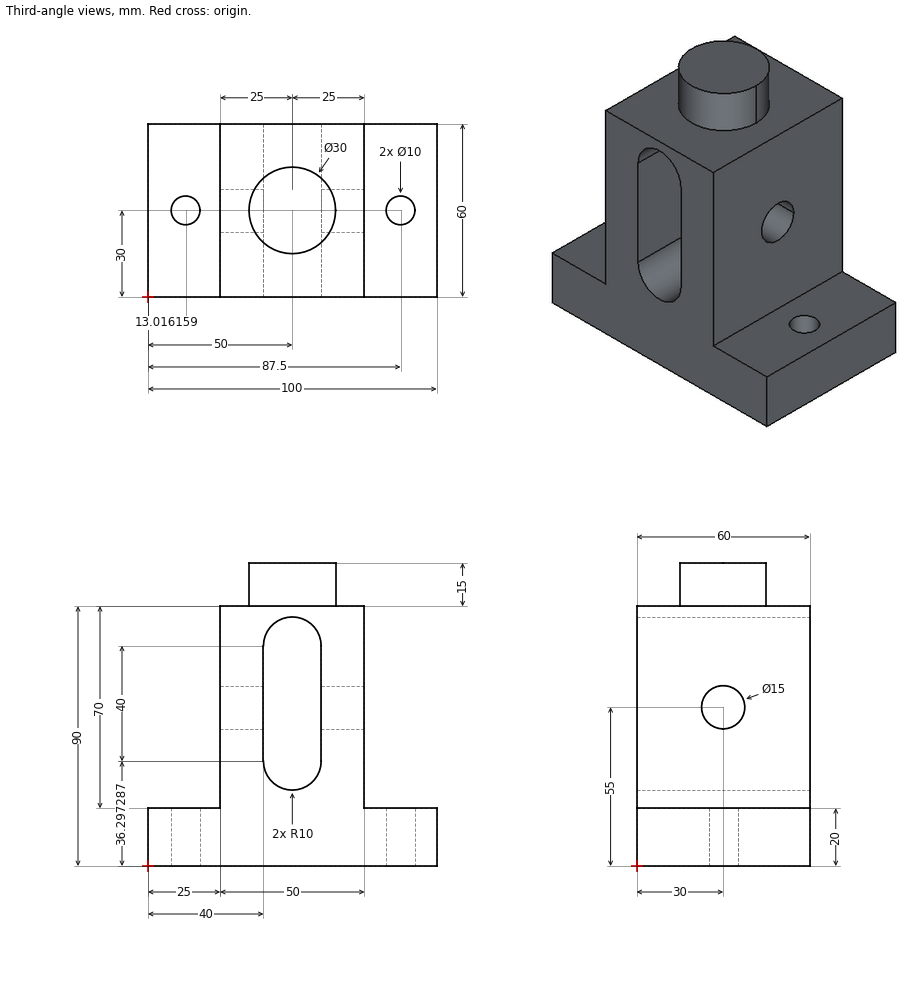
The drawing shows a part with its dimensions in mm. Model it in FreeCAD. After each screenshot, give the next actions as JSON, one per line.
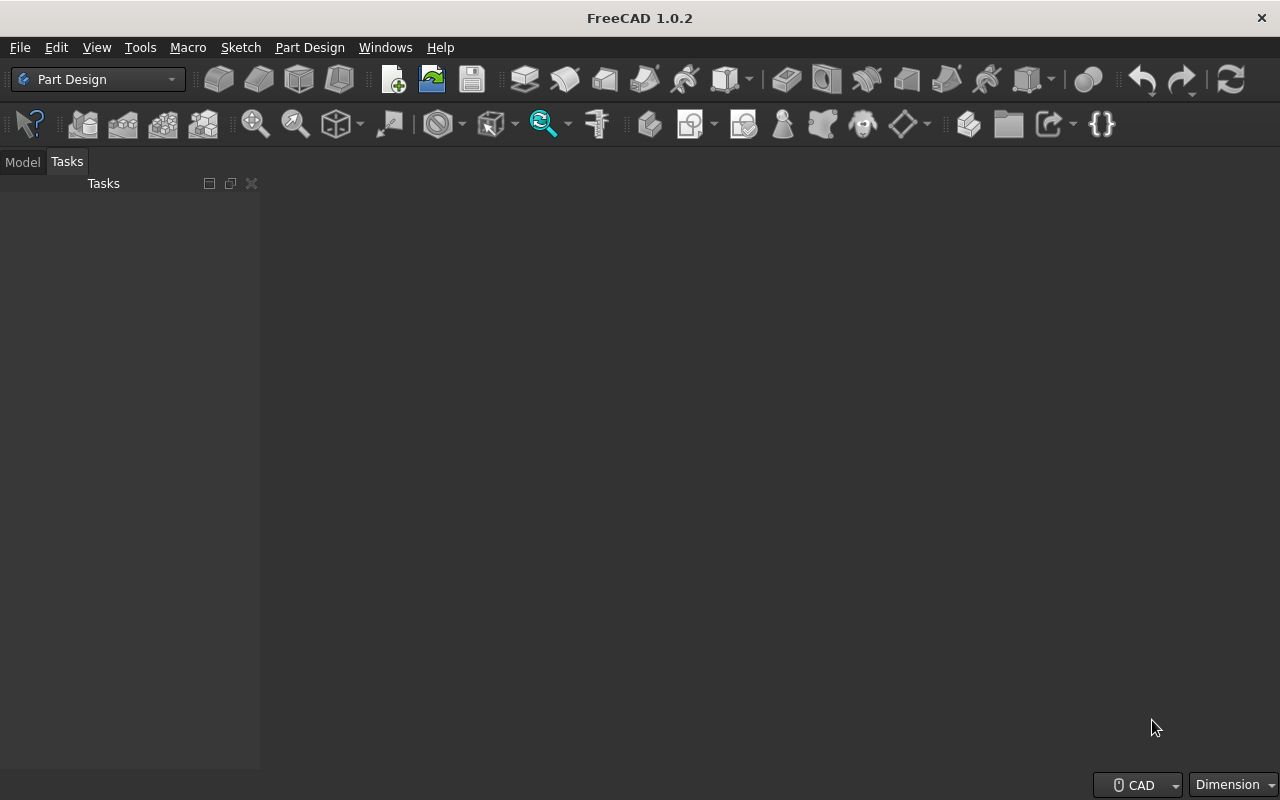
{"action": "left_click", "coordinate": [392, 80]}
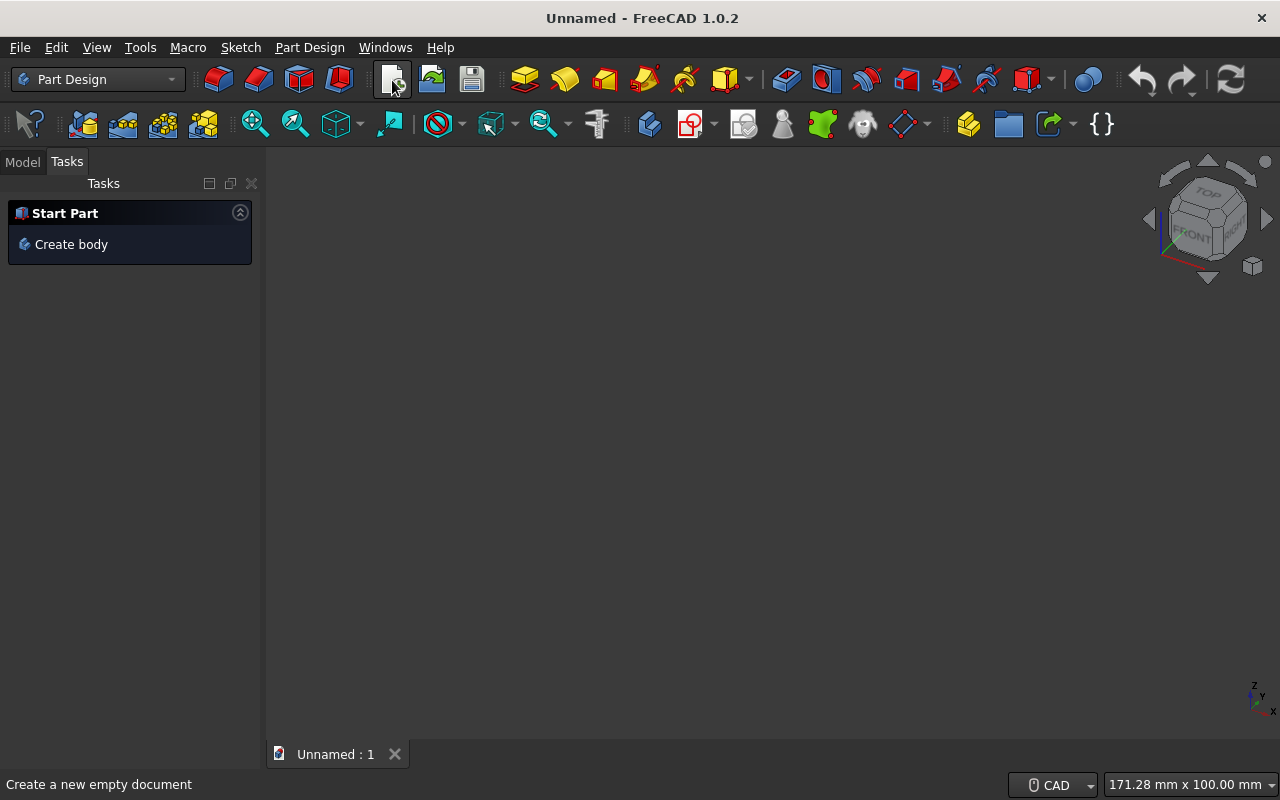
{"action": "left_click", "coordinate": [690, 124]}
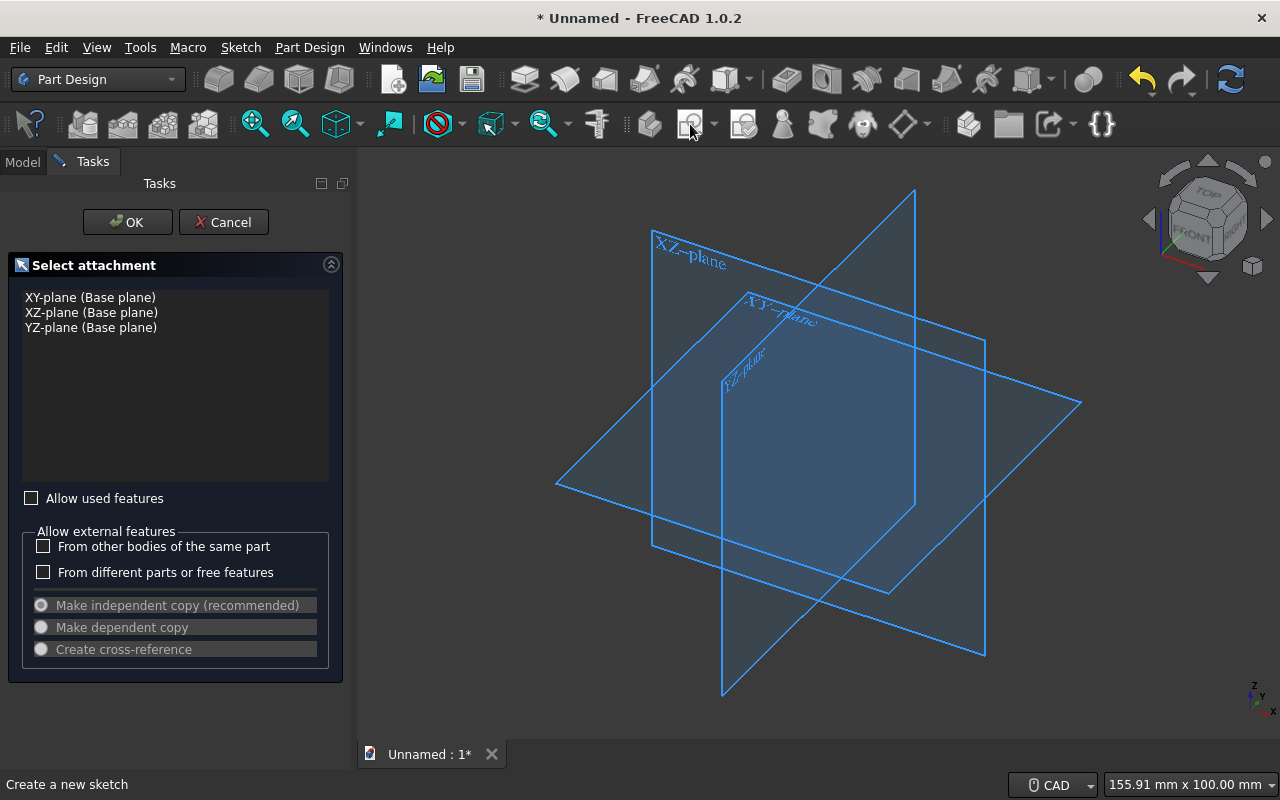
{"action": "left_click", "coordinate": [82, 298]}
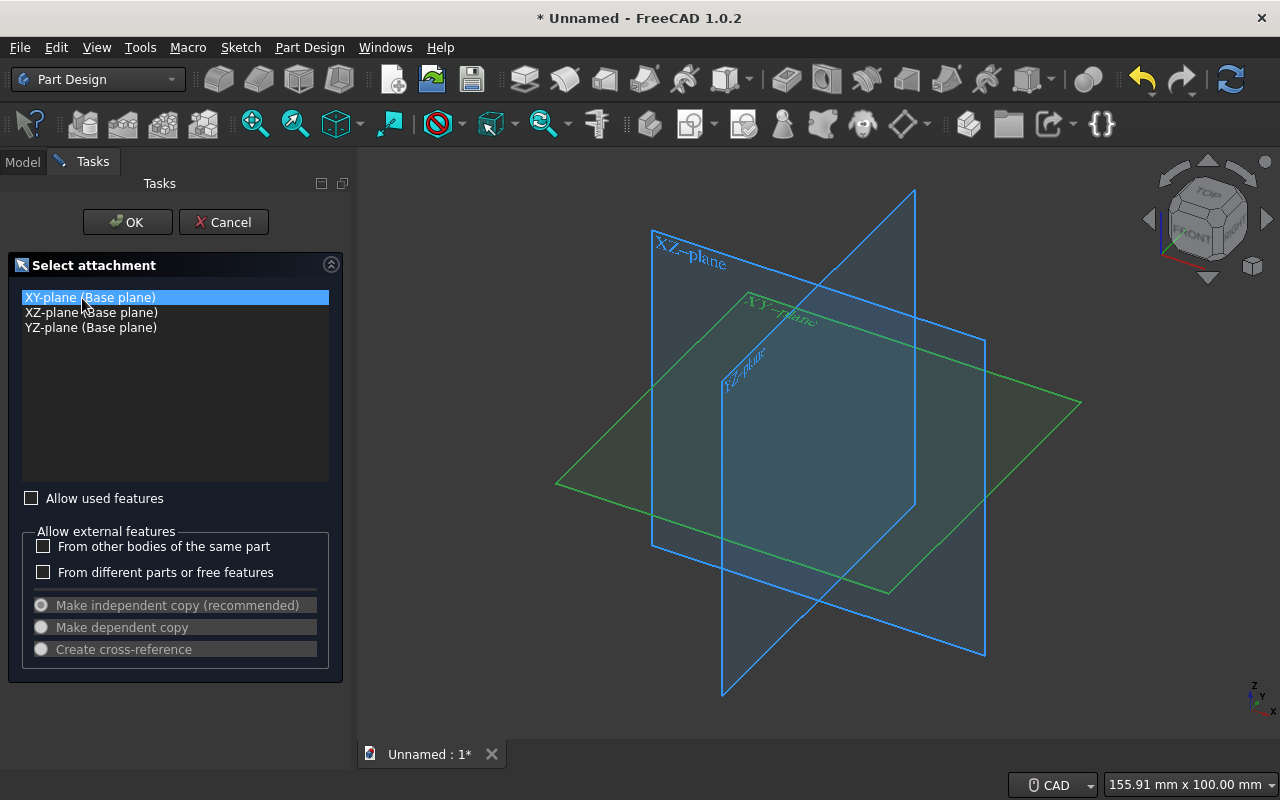
{"action": "left_click", "coordinate": [128, 222]}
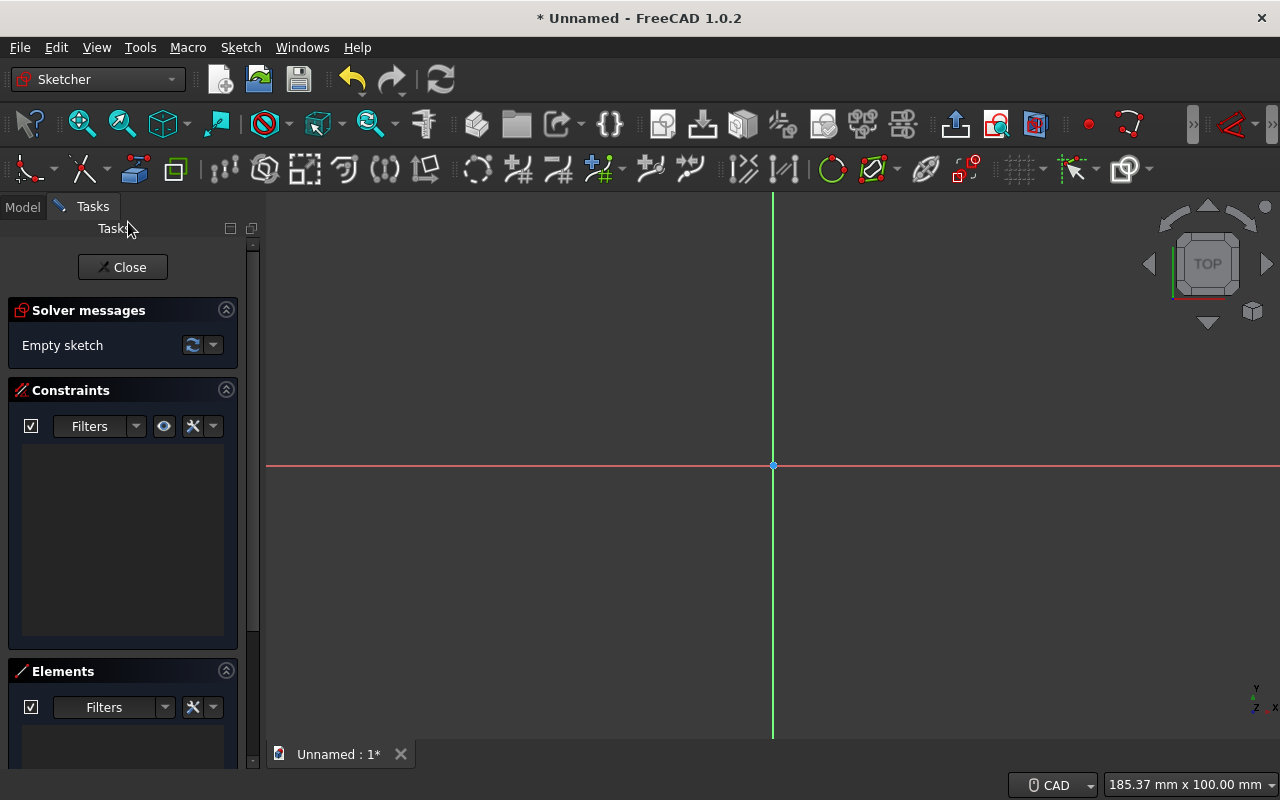
{"action": "scroll", "coordinate": [294, 711], "scroll_direction": "down", "scroll_amount": 2}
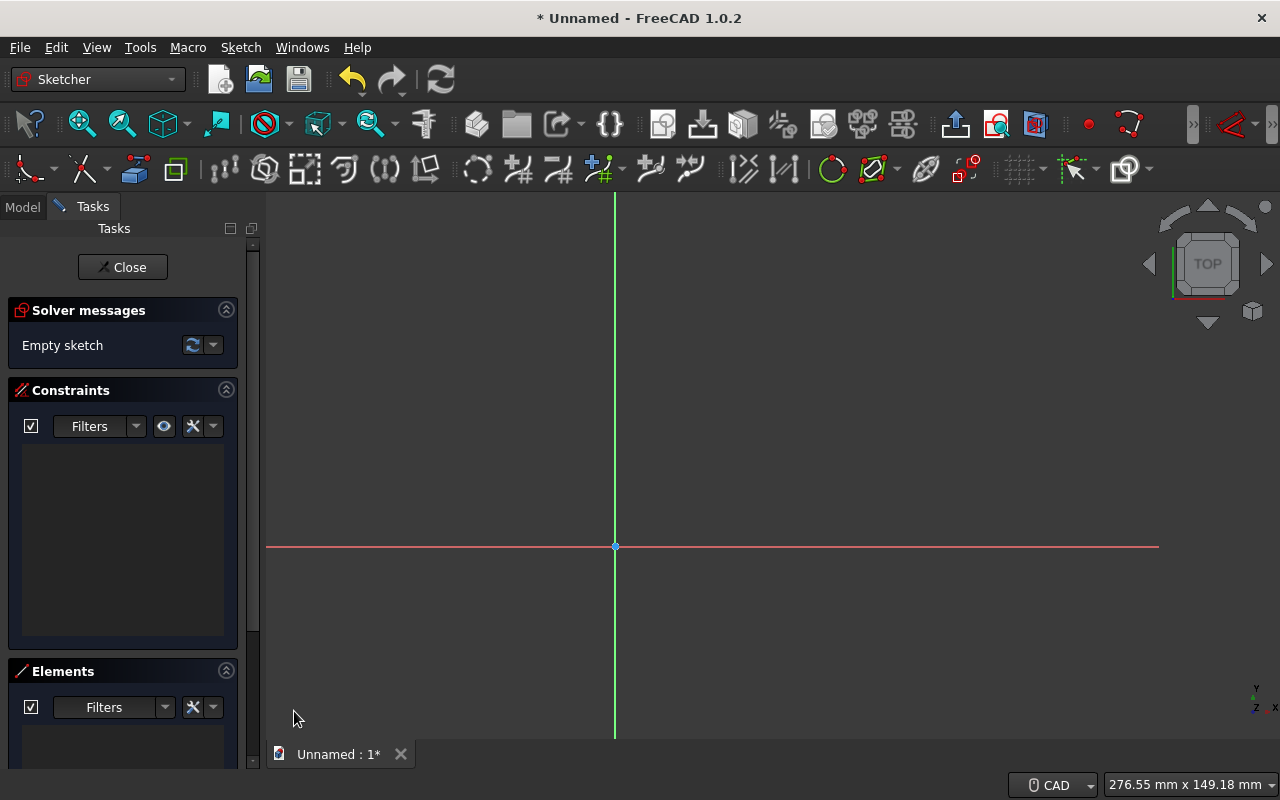
{"action": "scroll", "coordinate": [989, 378], "scroll_direction": "up", "scroll_amount": 2}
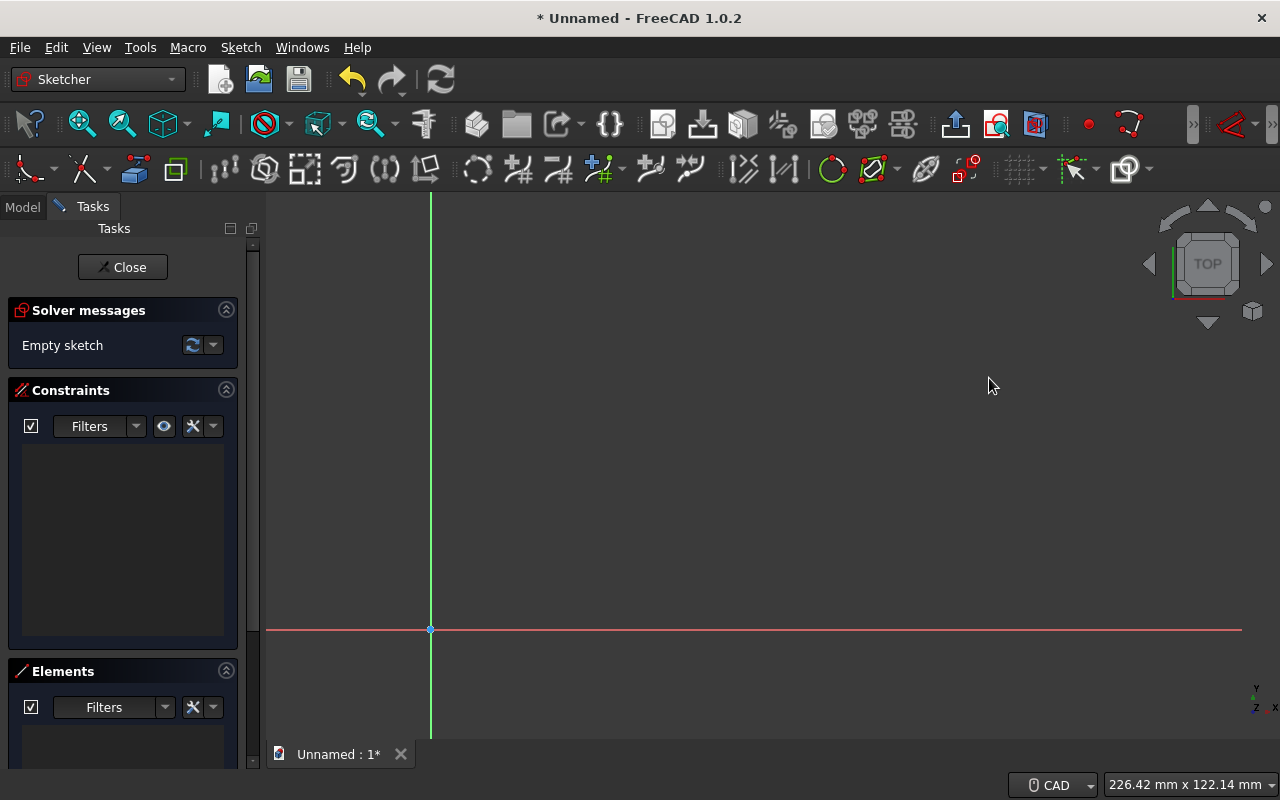
{"action": "key", "text": "g r"}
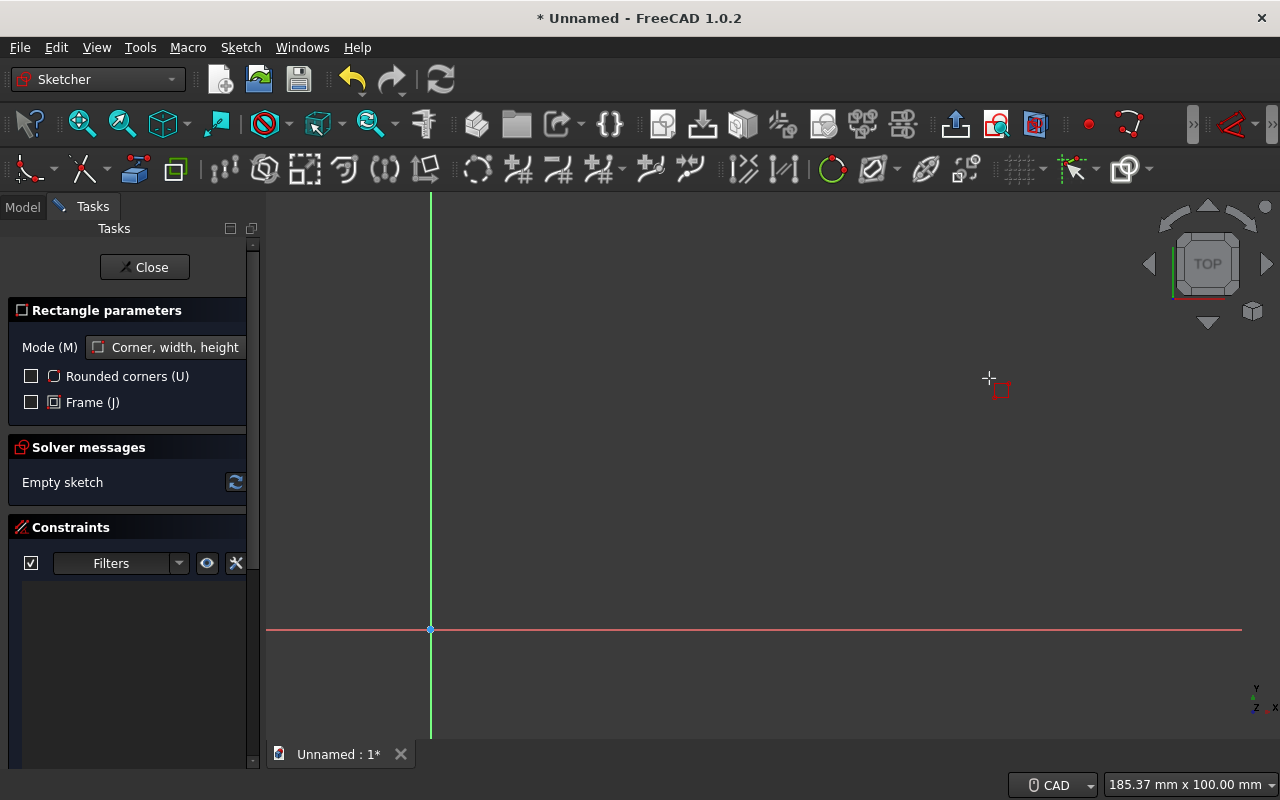
{"action": "left_click", "coordinate": [431, 630]}
{"action": "left_click", "coordinate": [978, 301]}
{"action": "key", "text": "Escape"}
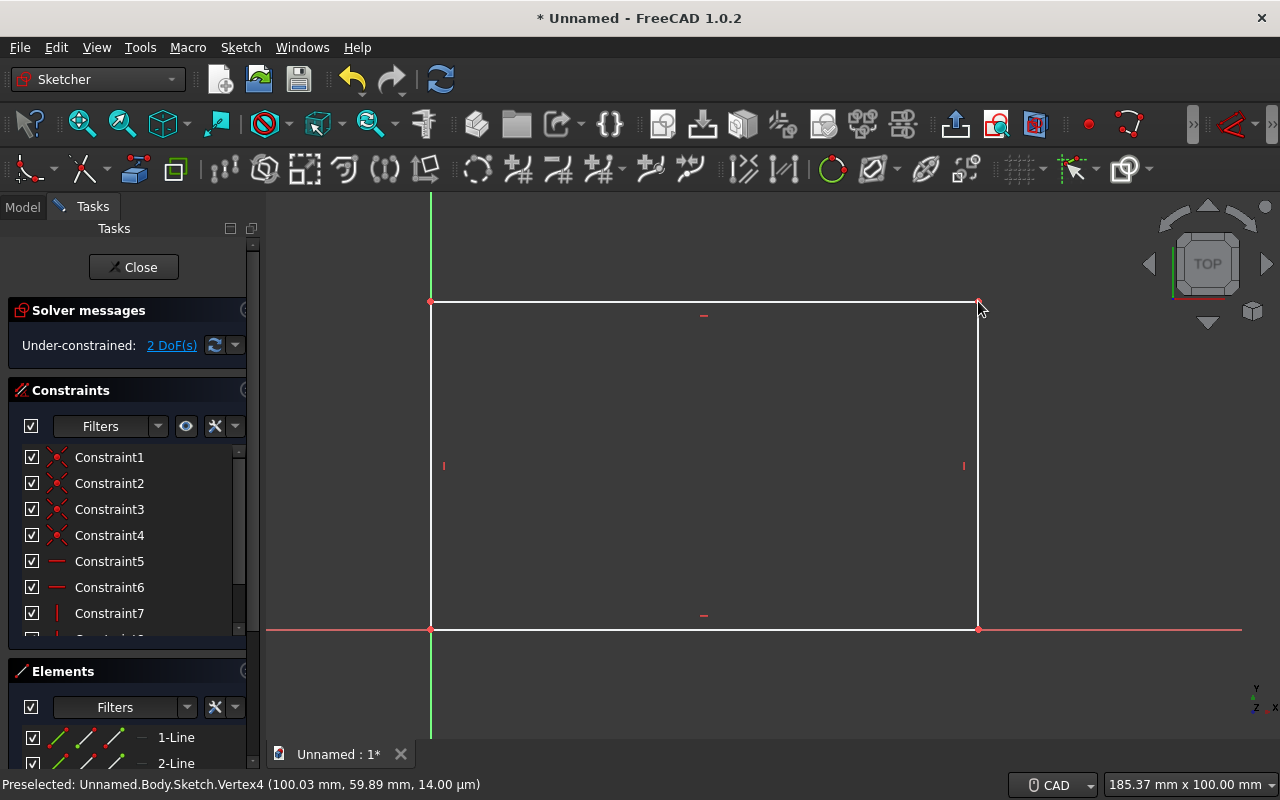
{"action": "left_click", "coordinate": [978, 531]}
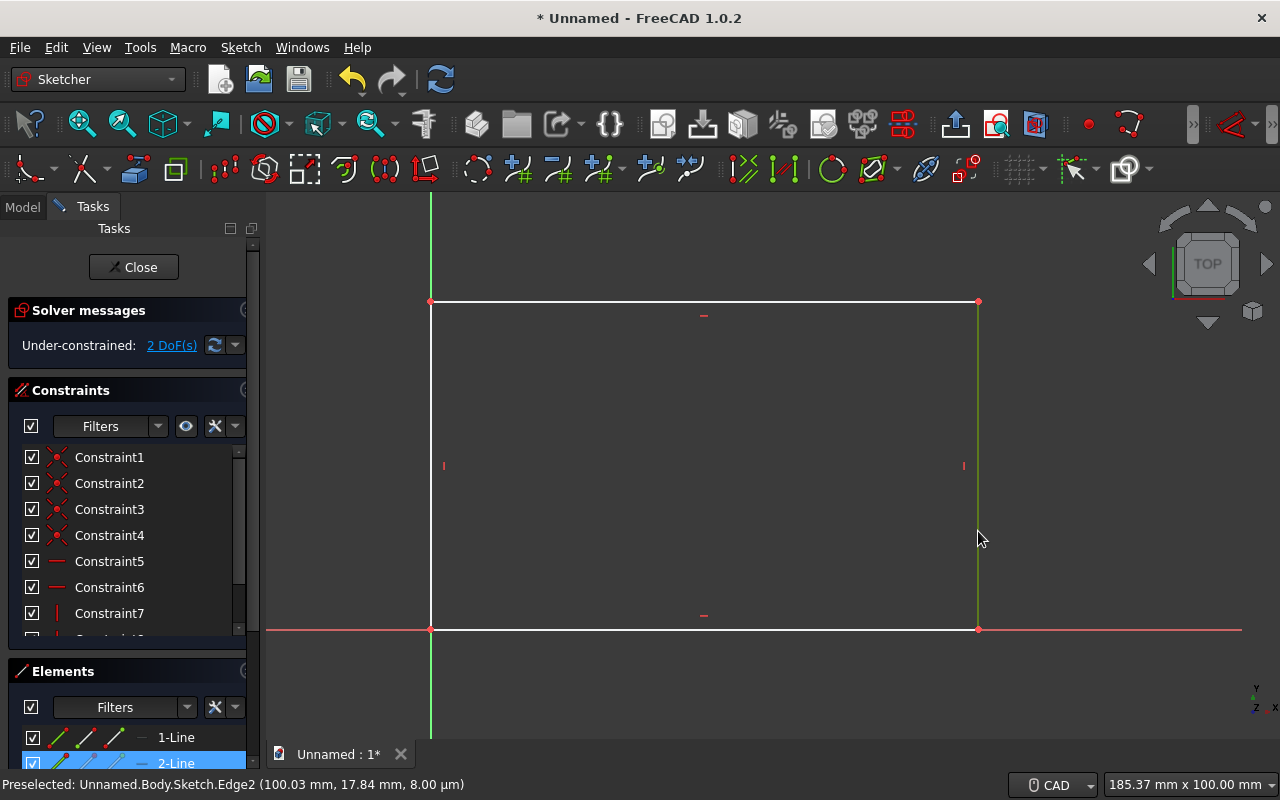
{"action": "key", "text": "i"}